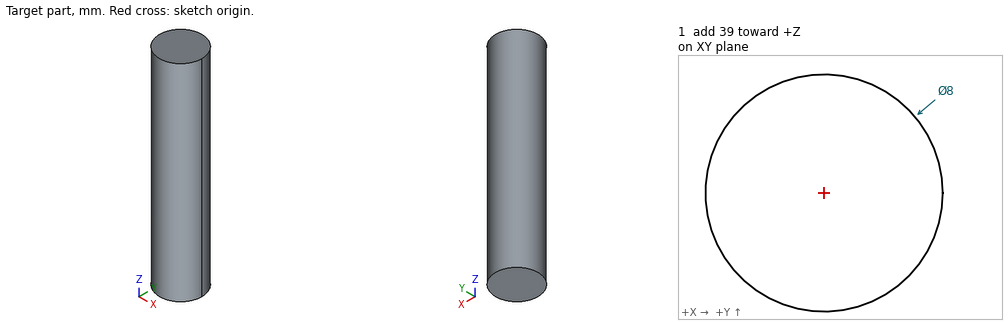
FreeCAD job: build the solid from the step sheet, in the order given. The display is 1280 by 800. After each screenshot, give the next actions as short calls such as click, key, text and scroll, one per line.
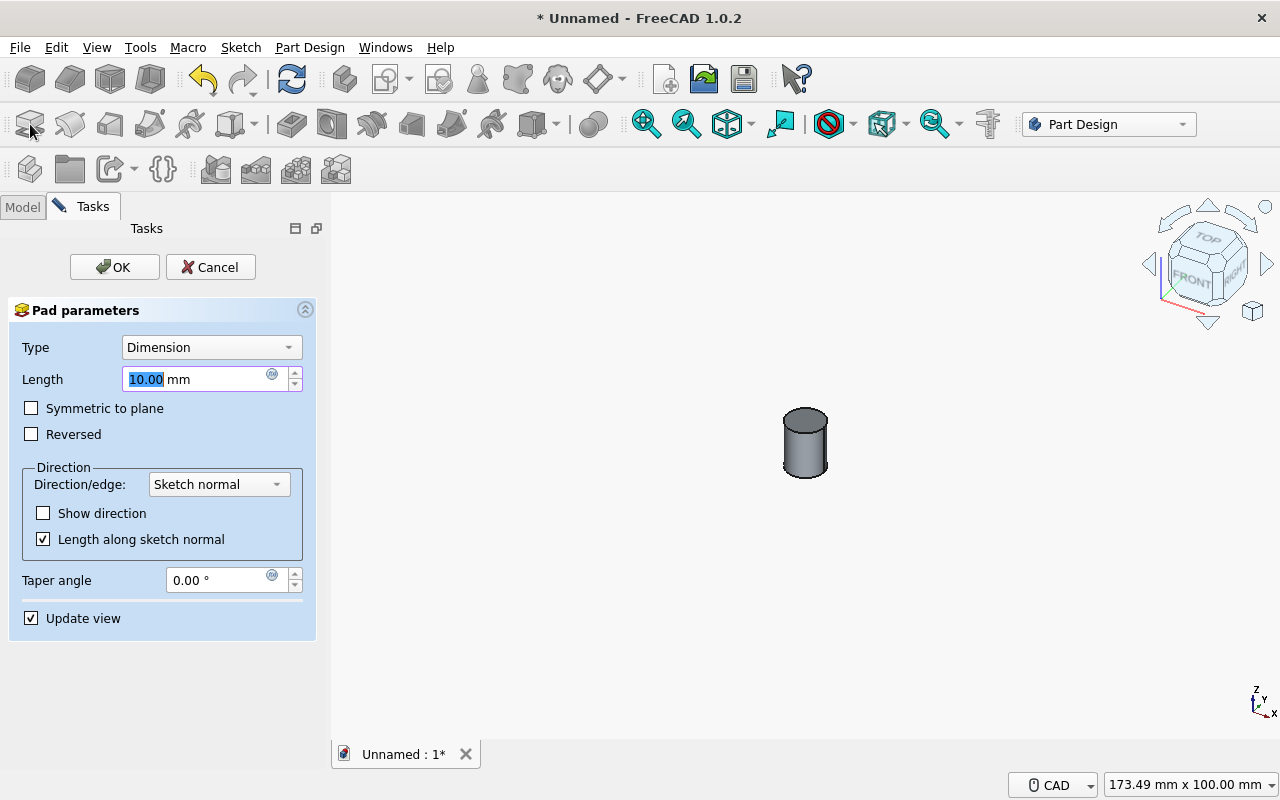
text(39)
key(Tab)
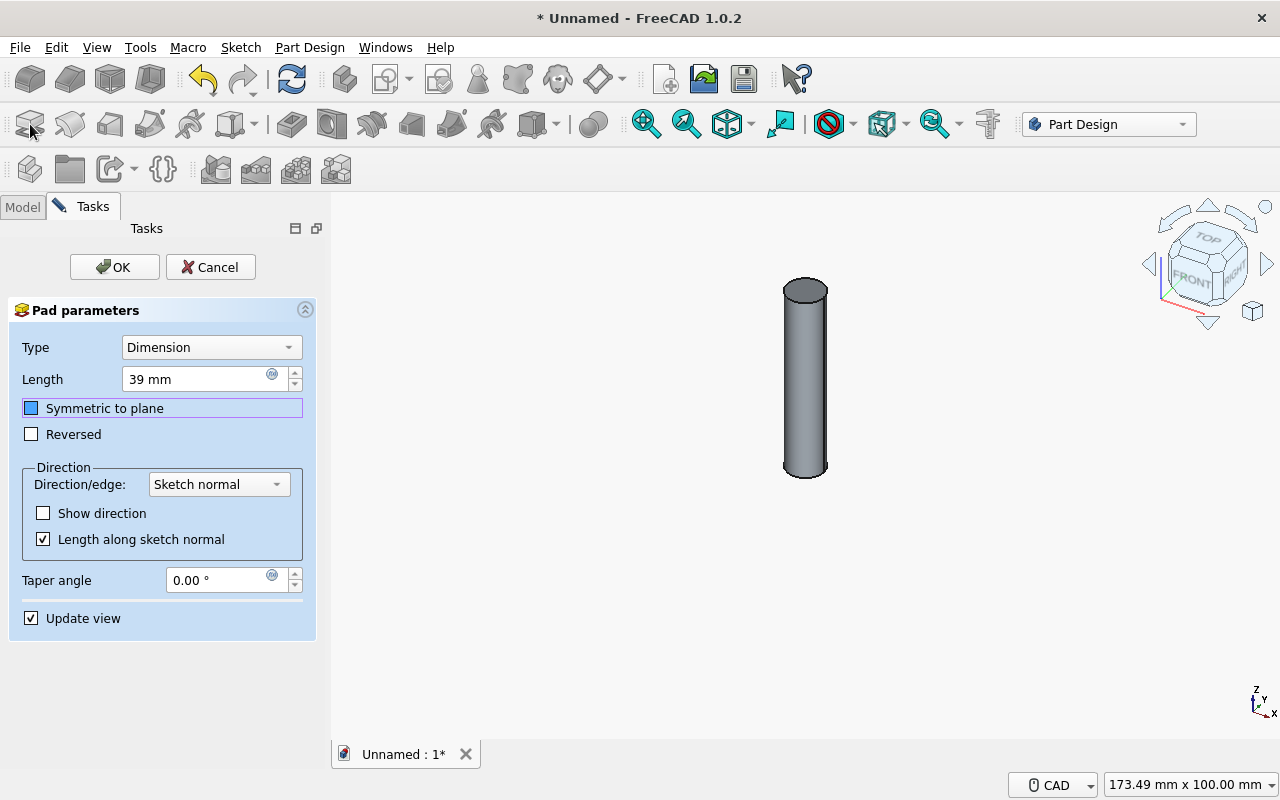
click(115, 267)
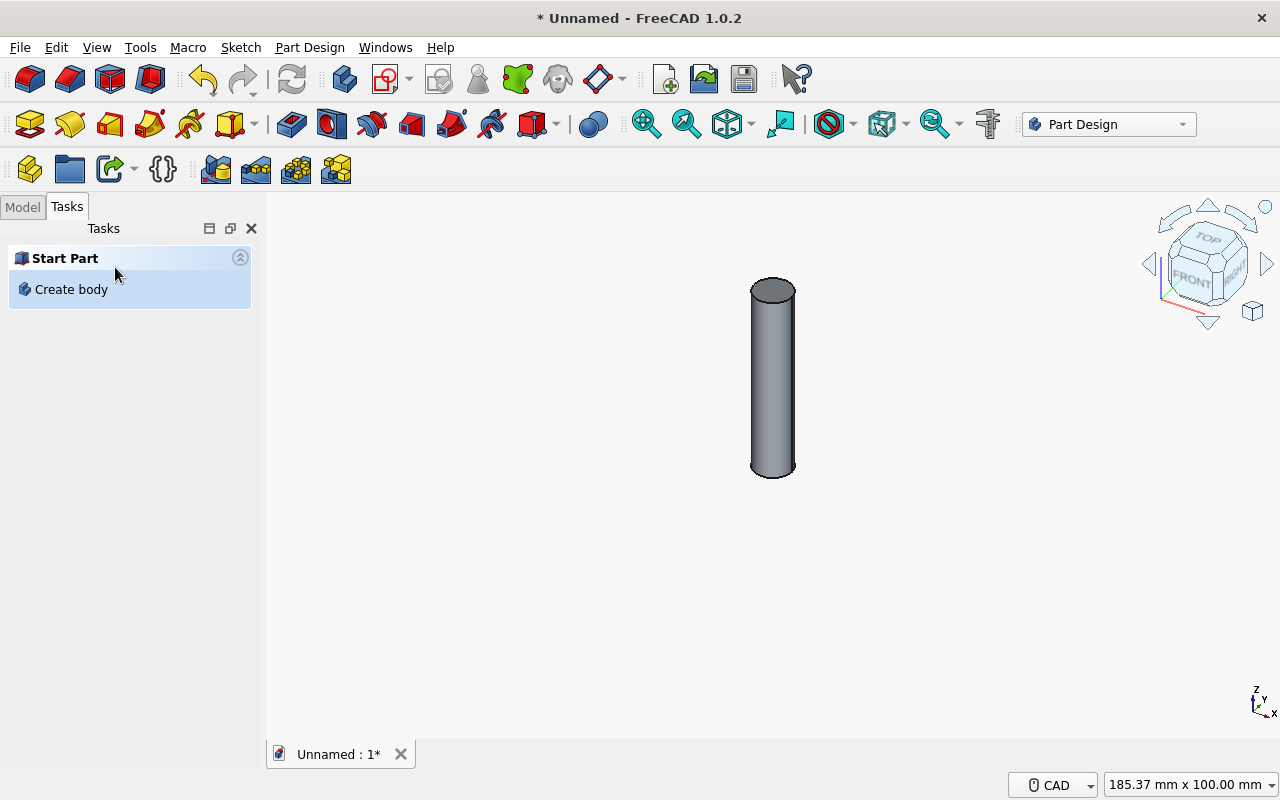
key(0)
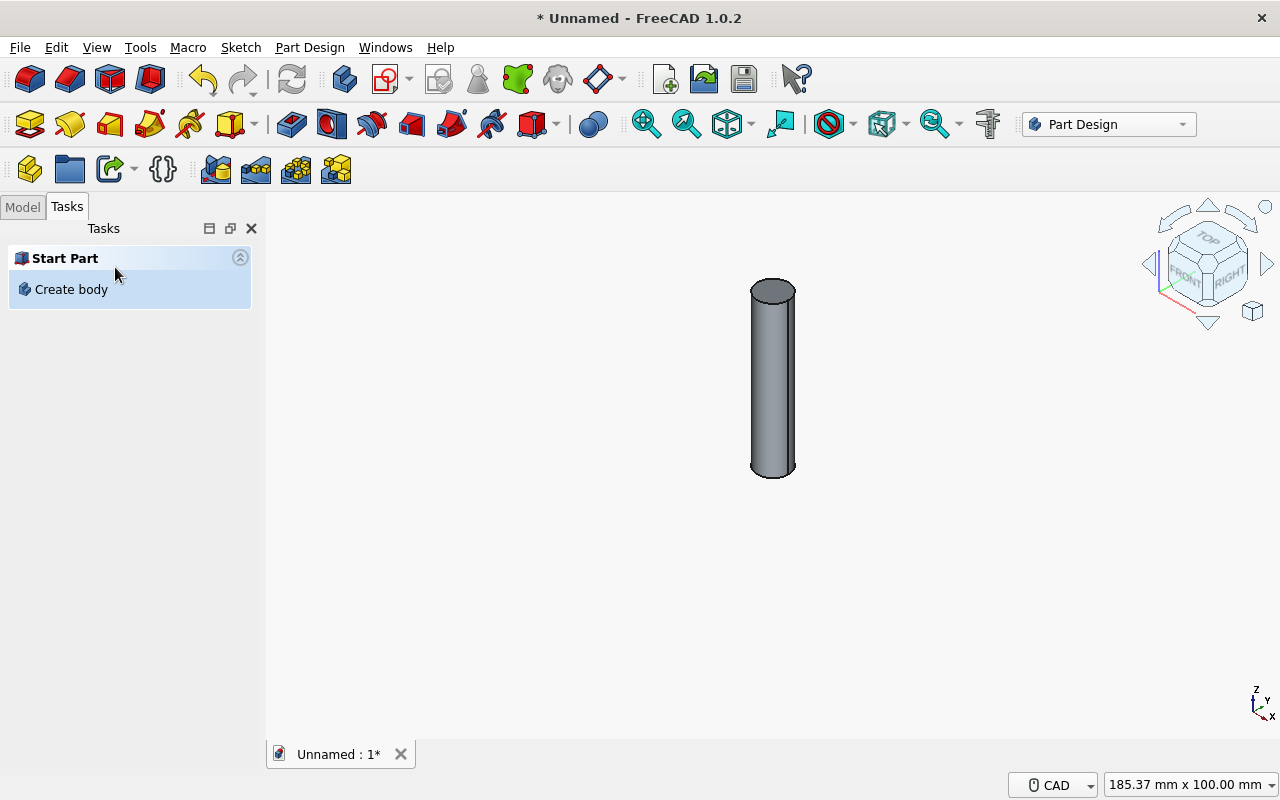
key(v)
key(f)